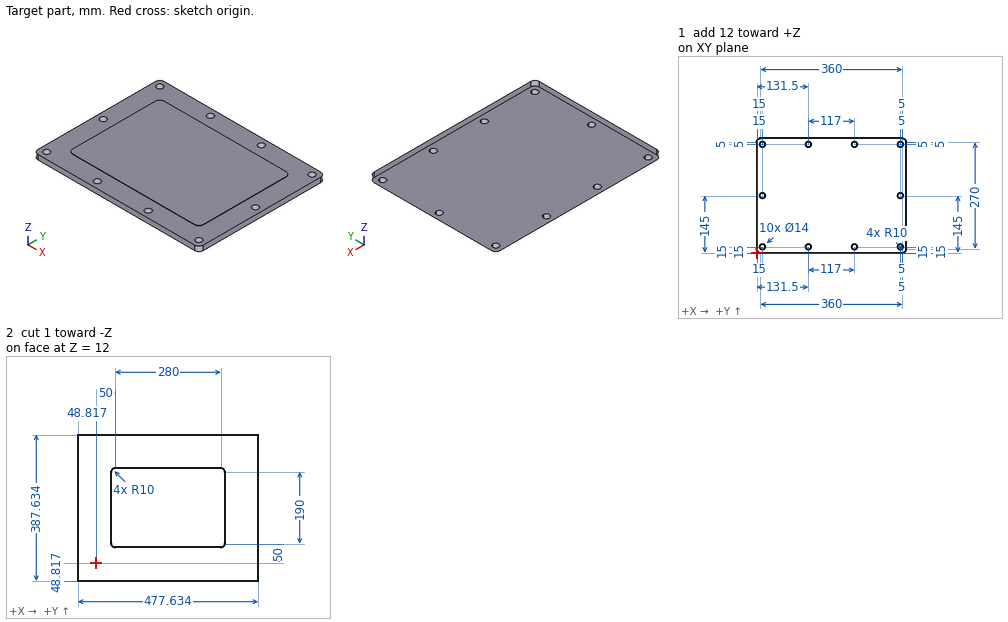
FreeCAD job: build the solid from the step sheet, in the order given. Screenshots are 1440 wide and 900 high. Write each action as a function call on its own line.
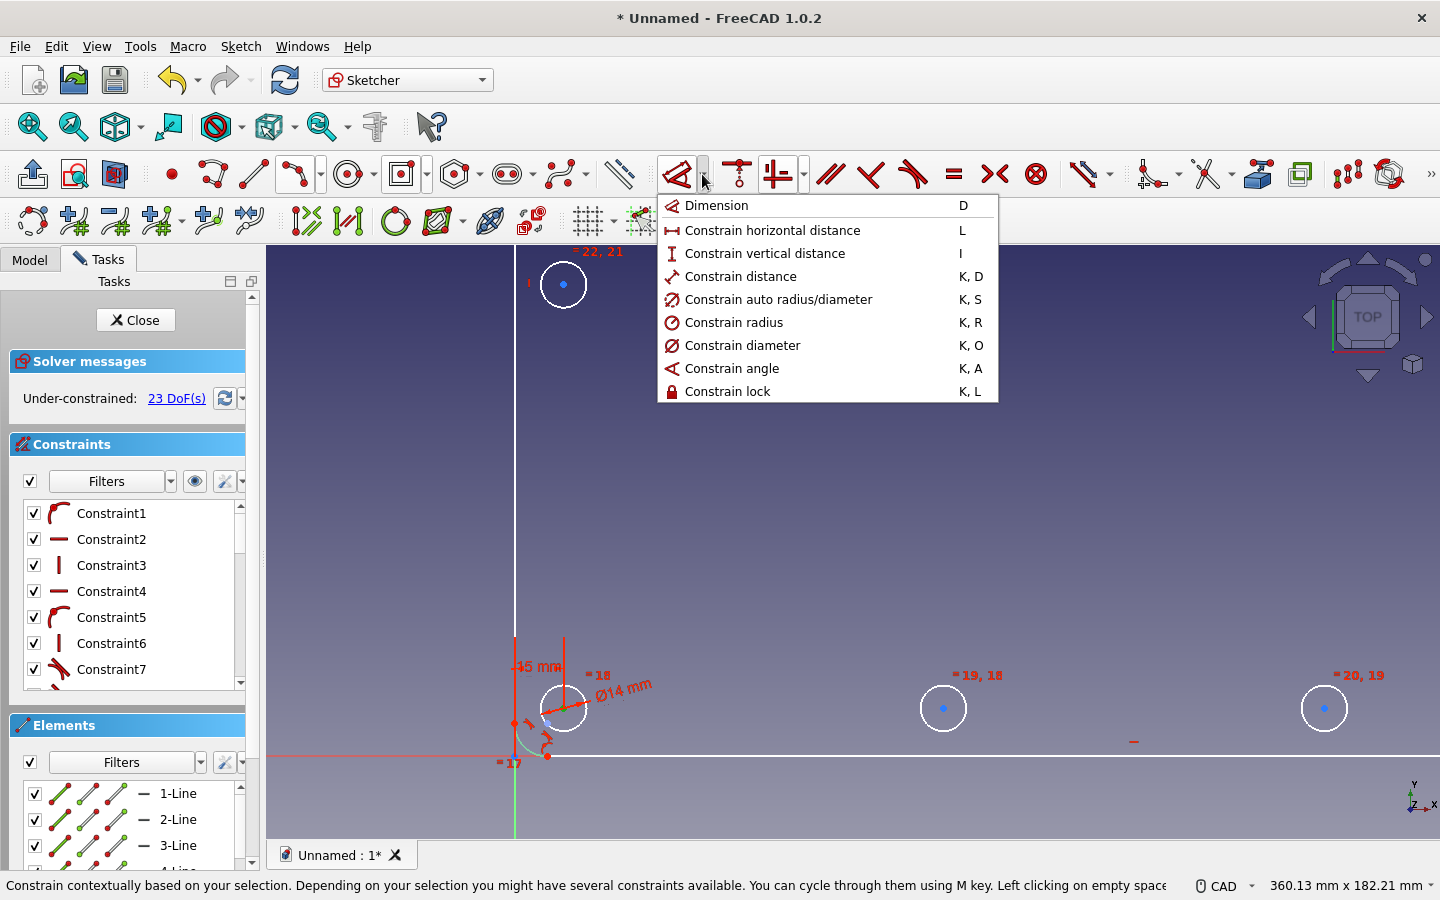
click(828, 254)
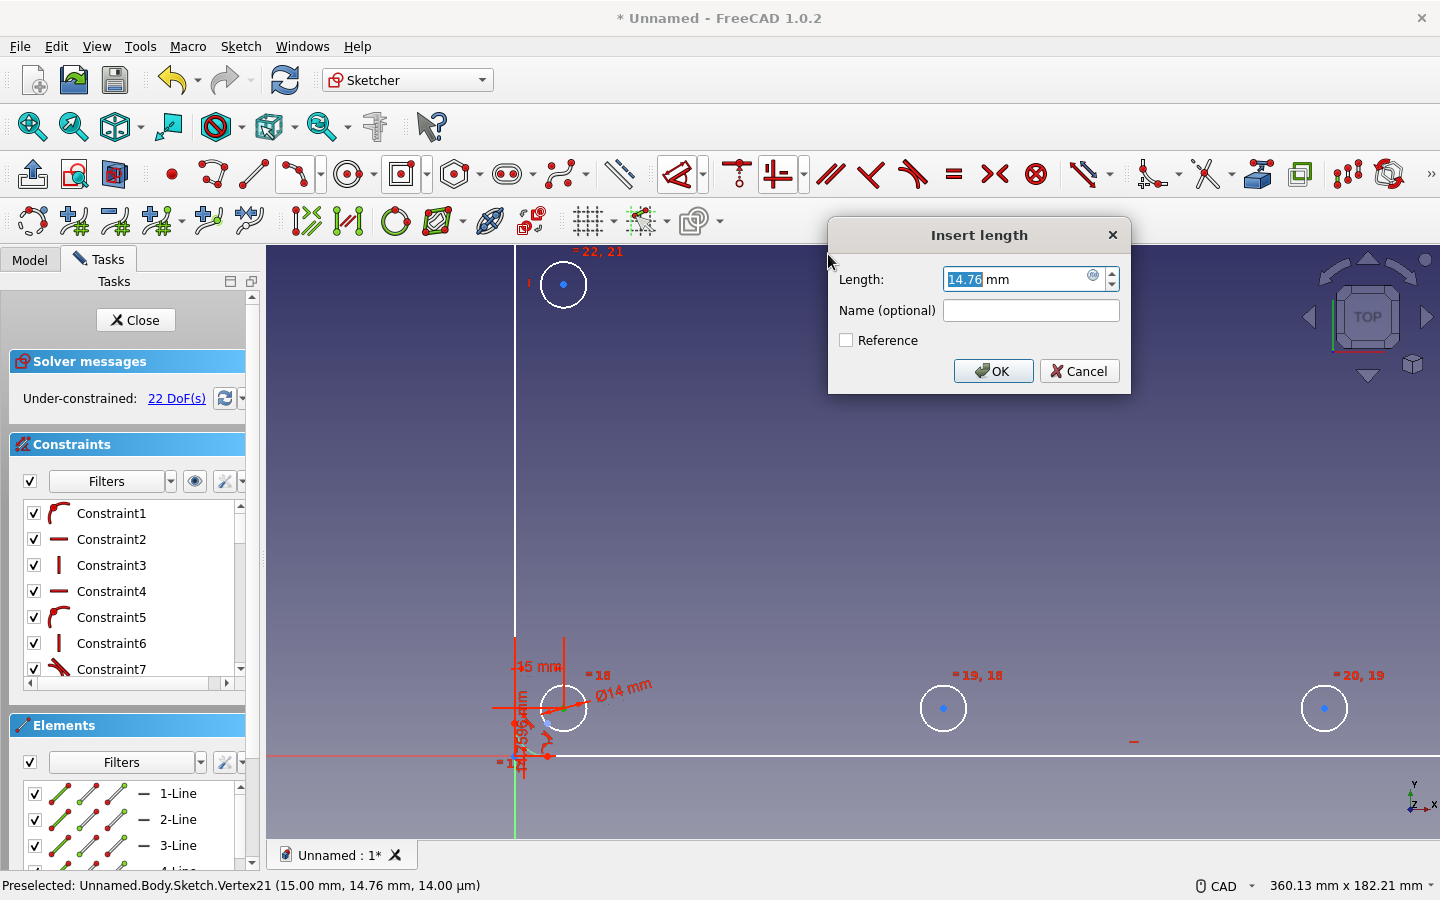
text(15)
key(Return)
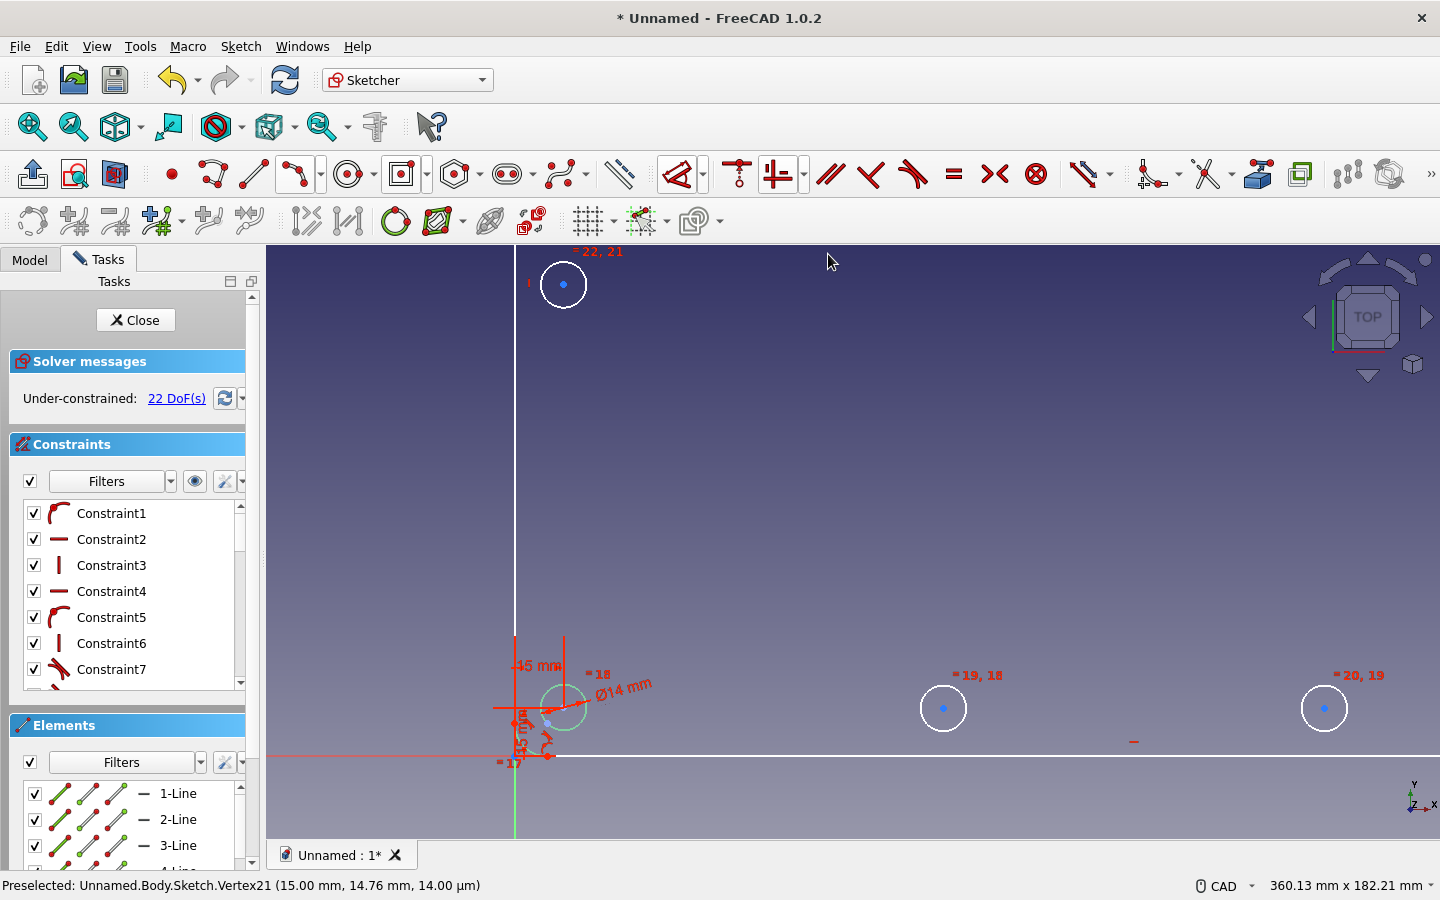
click(943, 708)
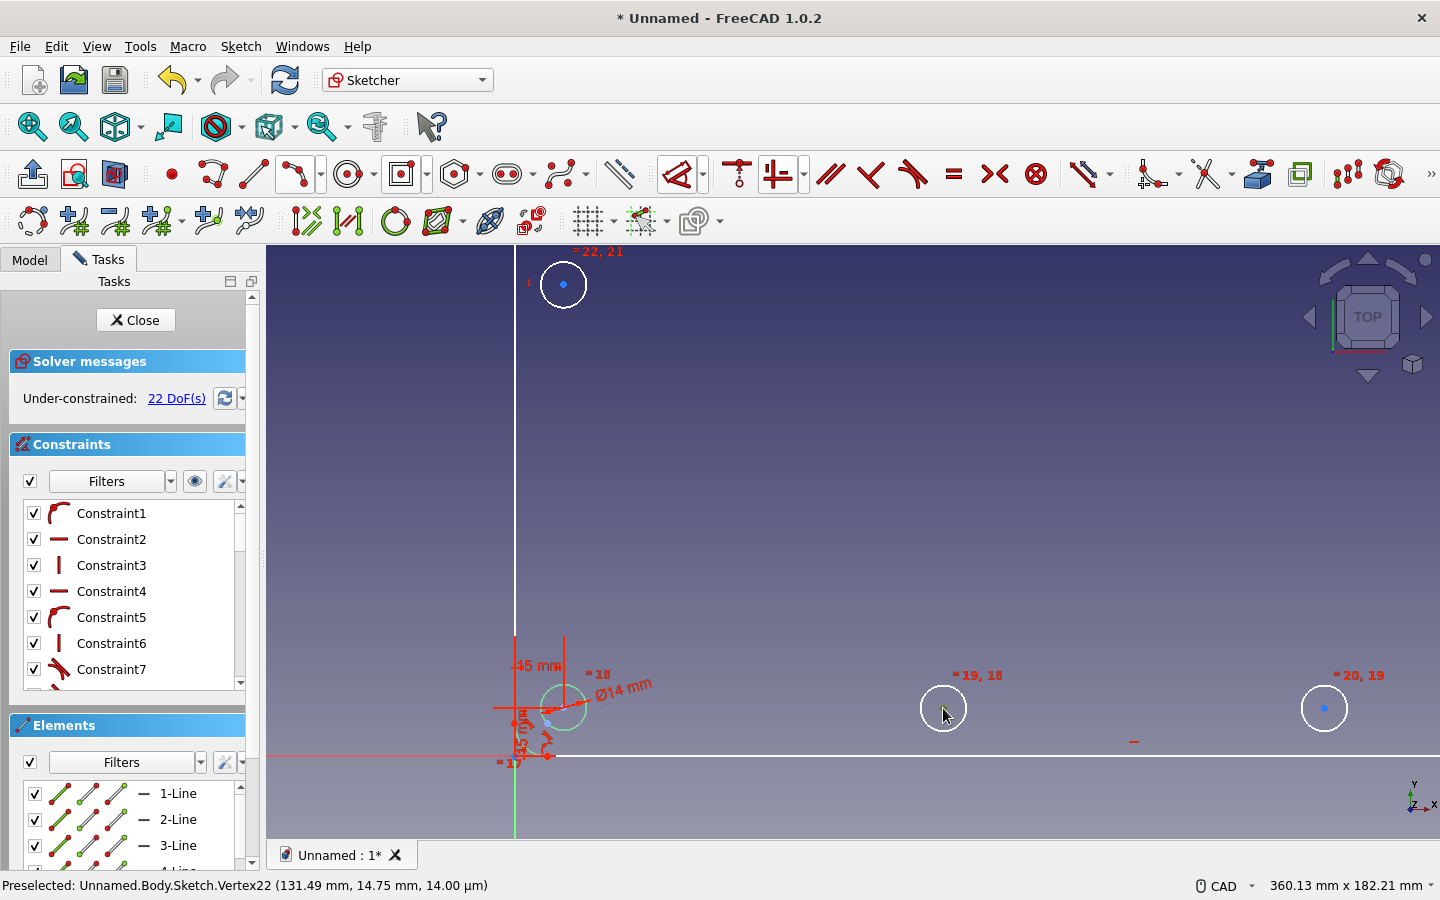
click(702, 174)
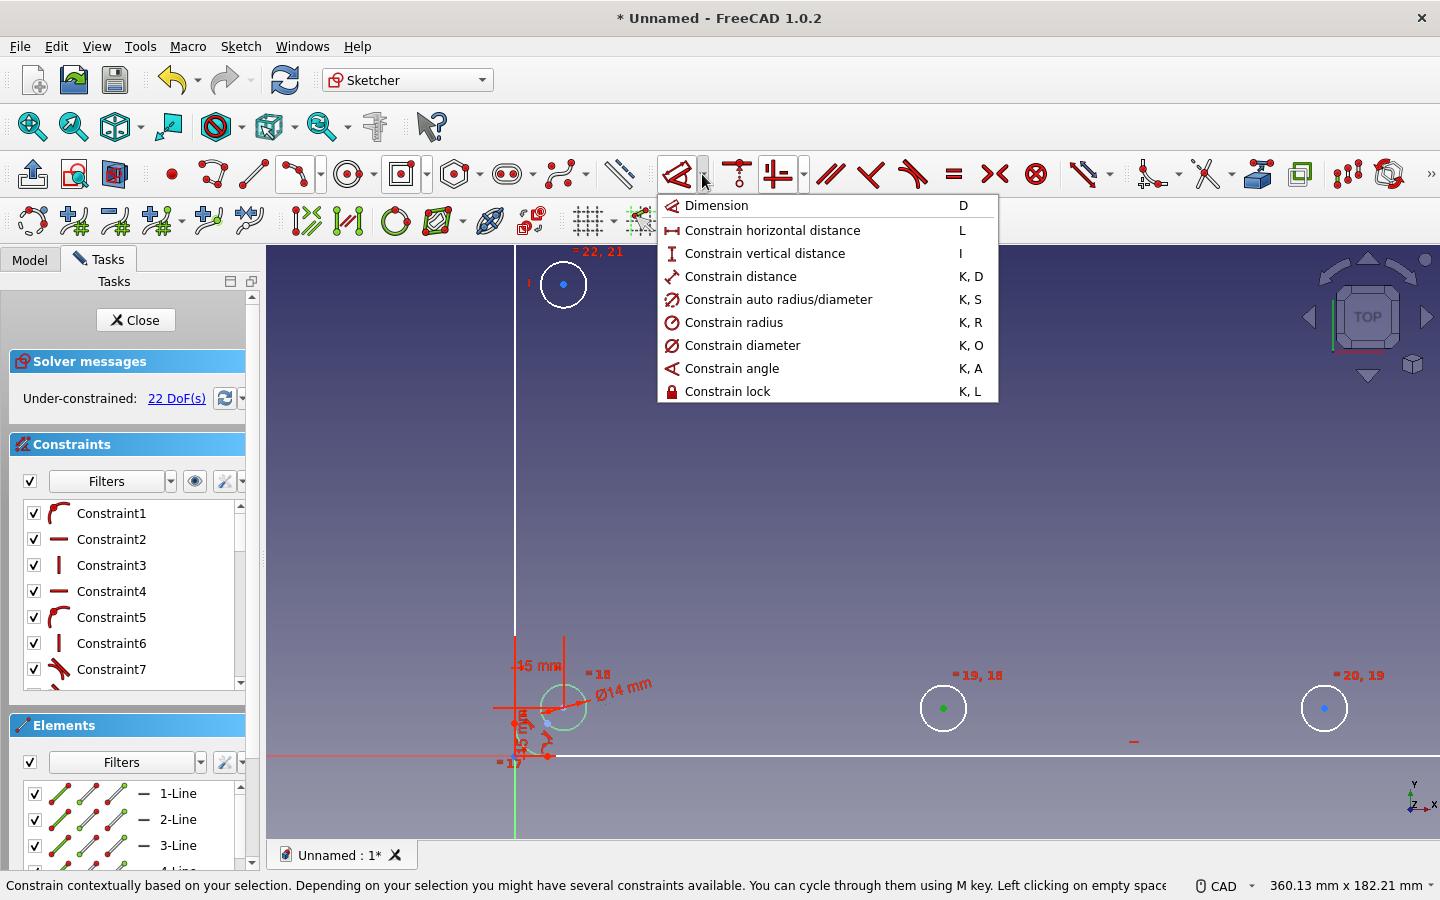
click(828, 254)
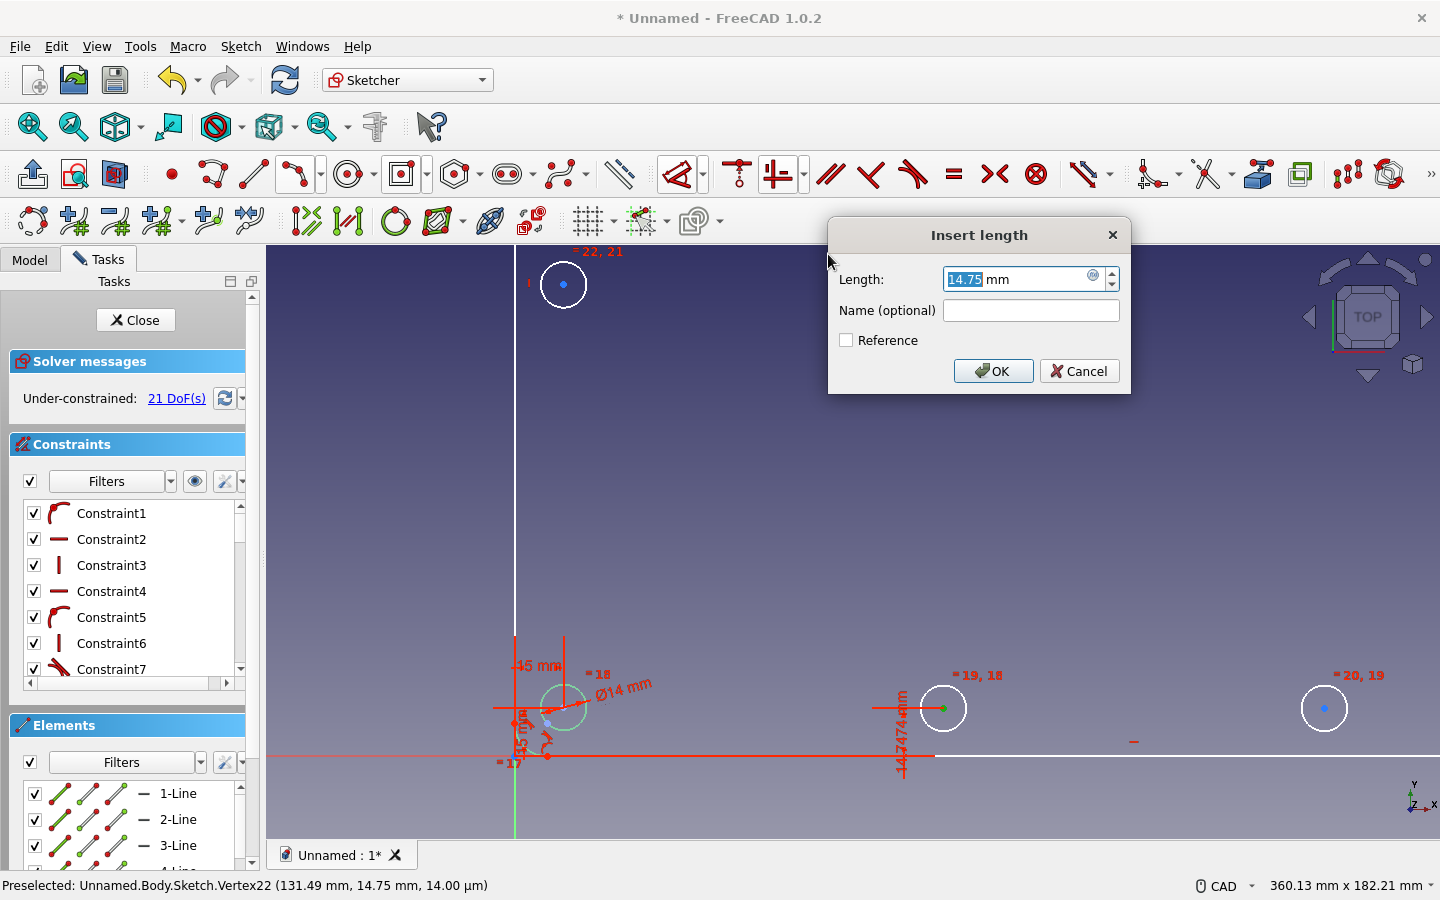
text(15)
key(Return)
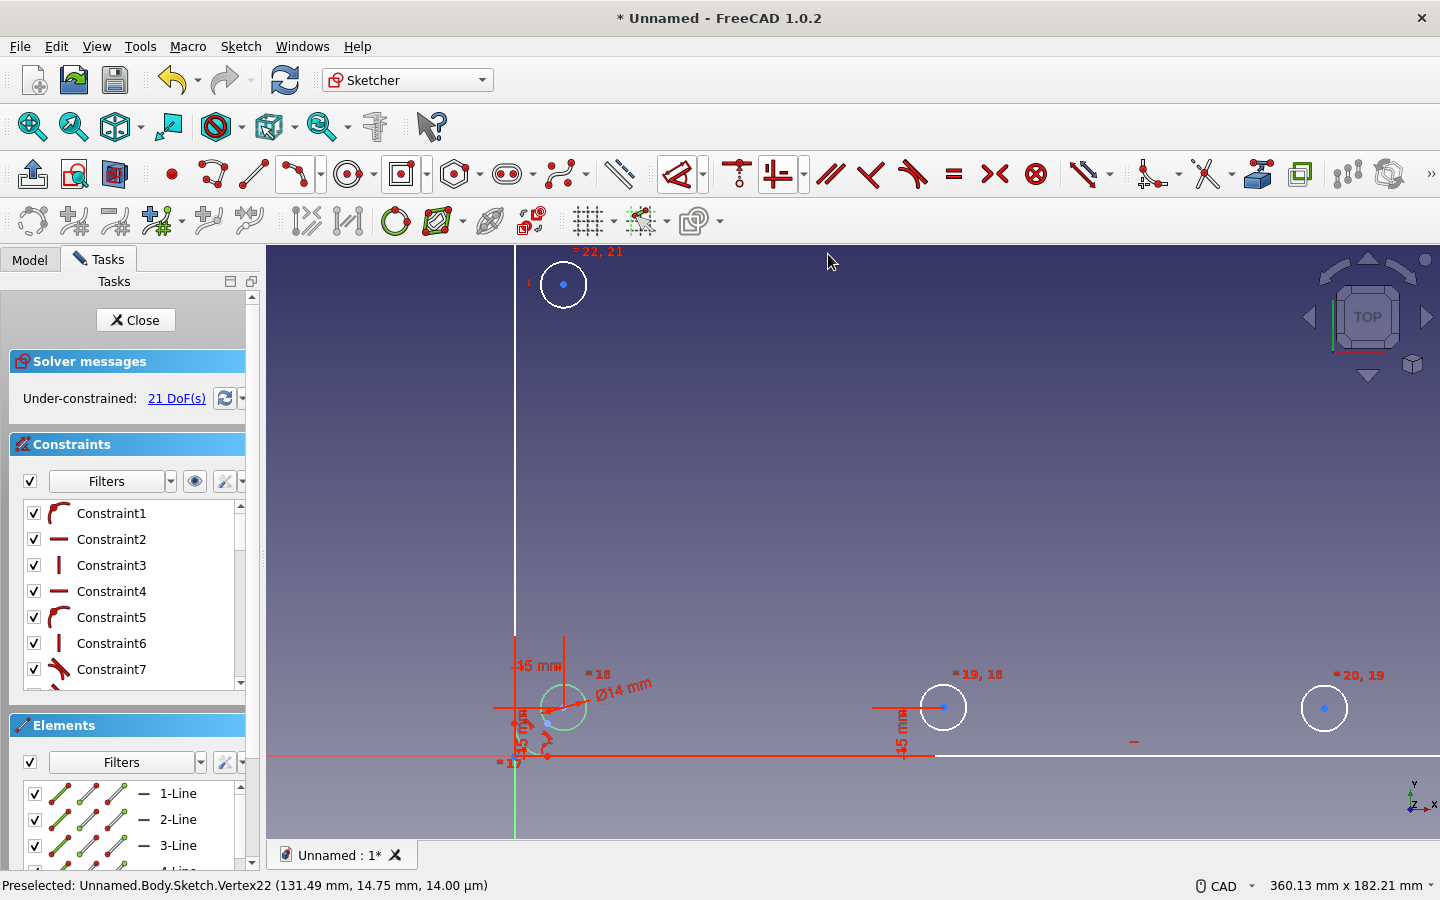
scroll(581, 692, down, 5)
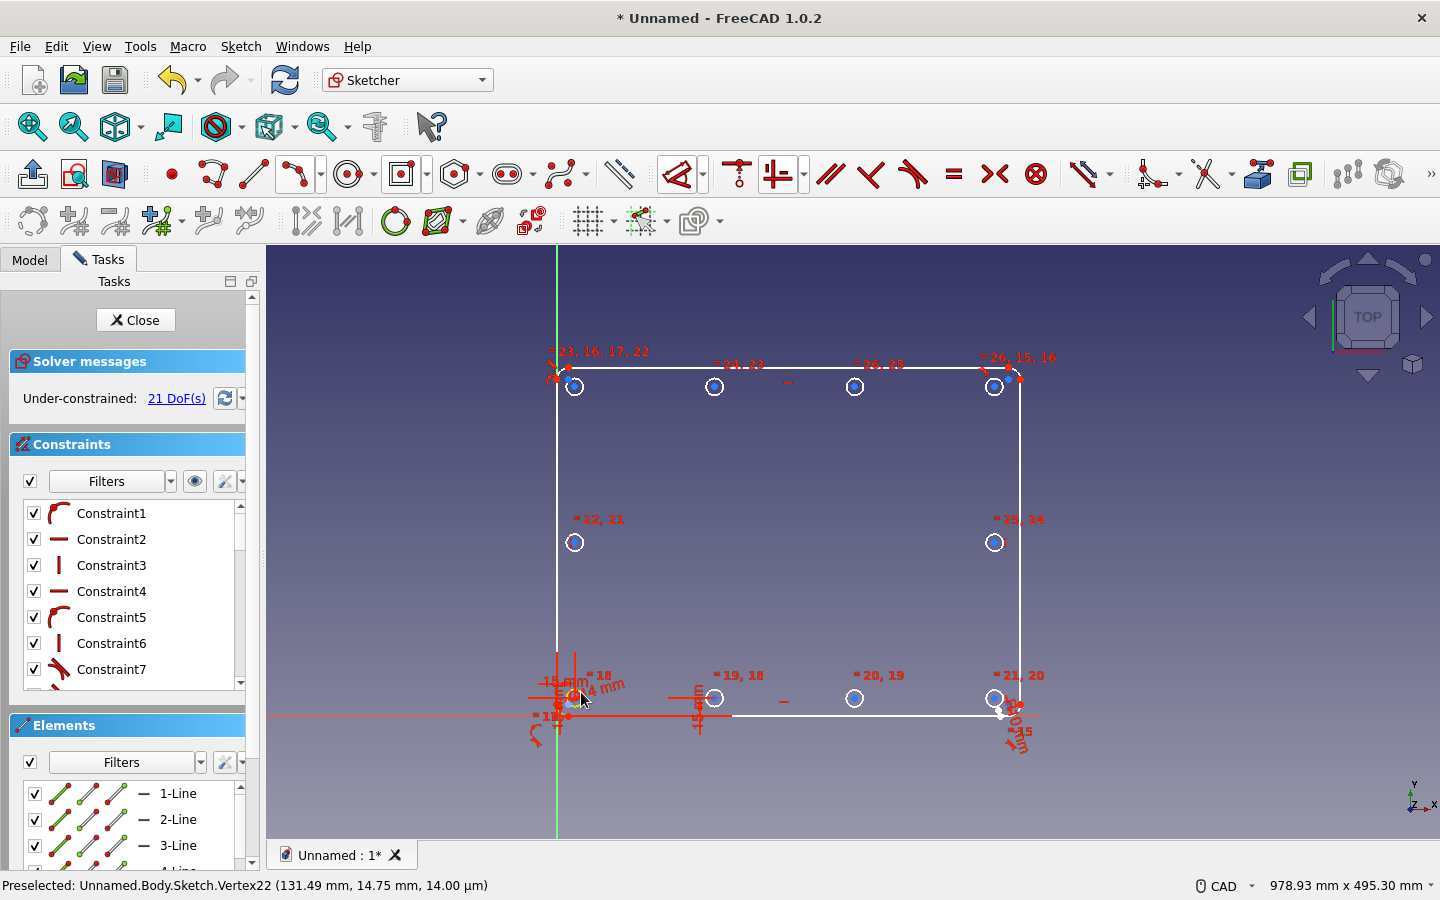
scroll(855, 698, up, 4)